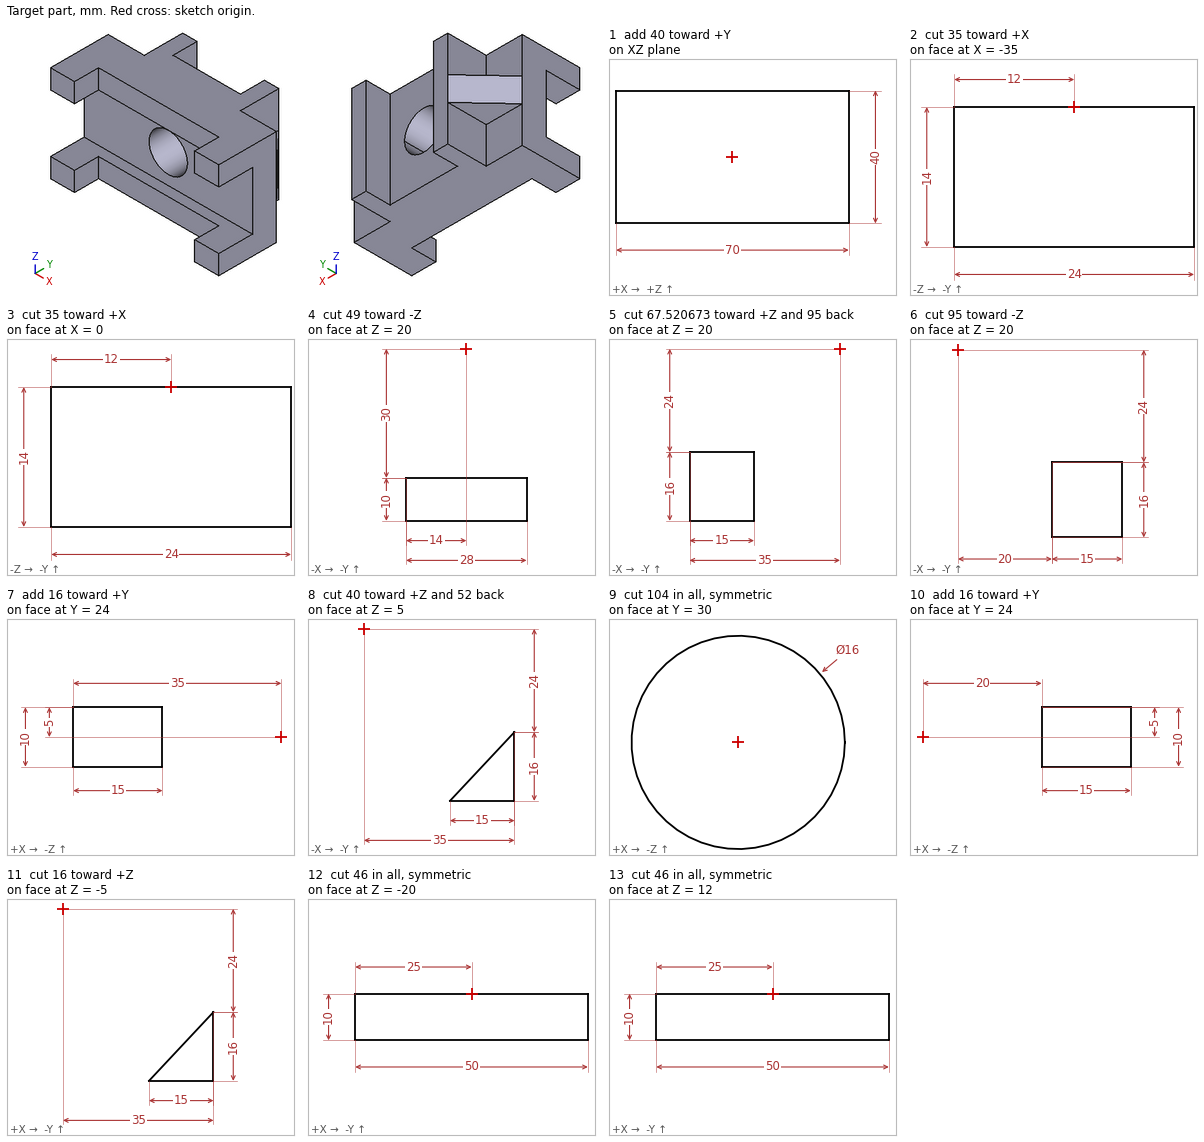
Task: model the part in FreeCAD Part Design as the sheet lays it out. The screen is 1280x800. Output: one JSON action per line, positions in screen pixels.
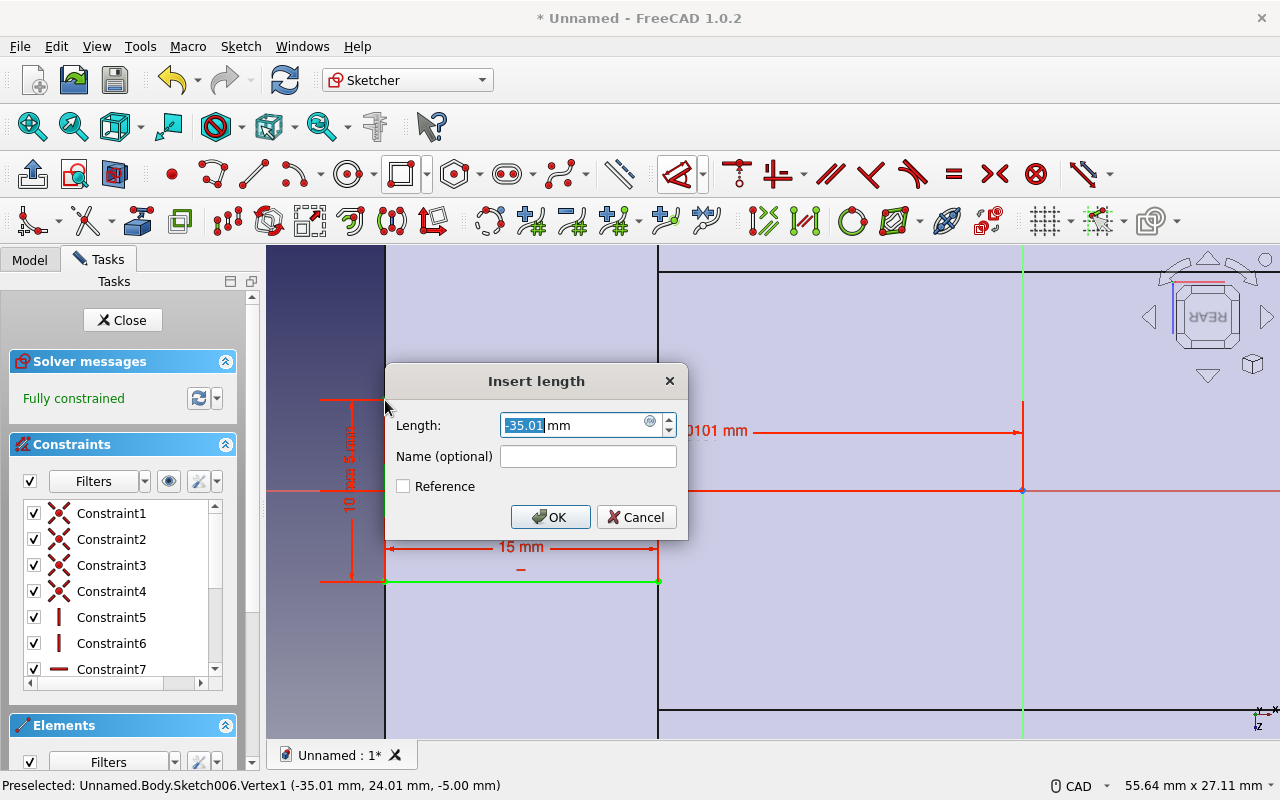
{"action": "type", "text": "-35"}
{"action": "key", "text": "Return"}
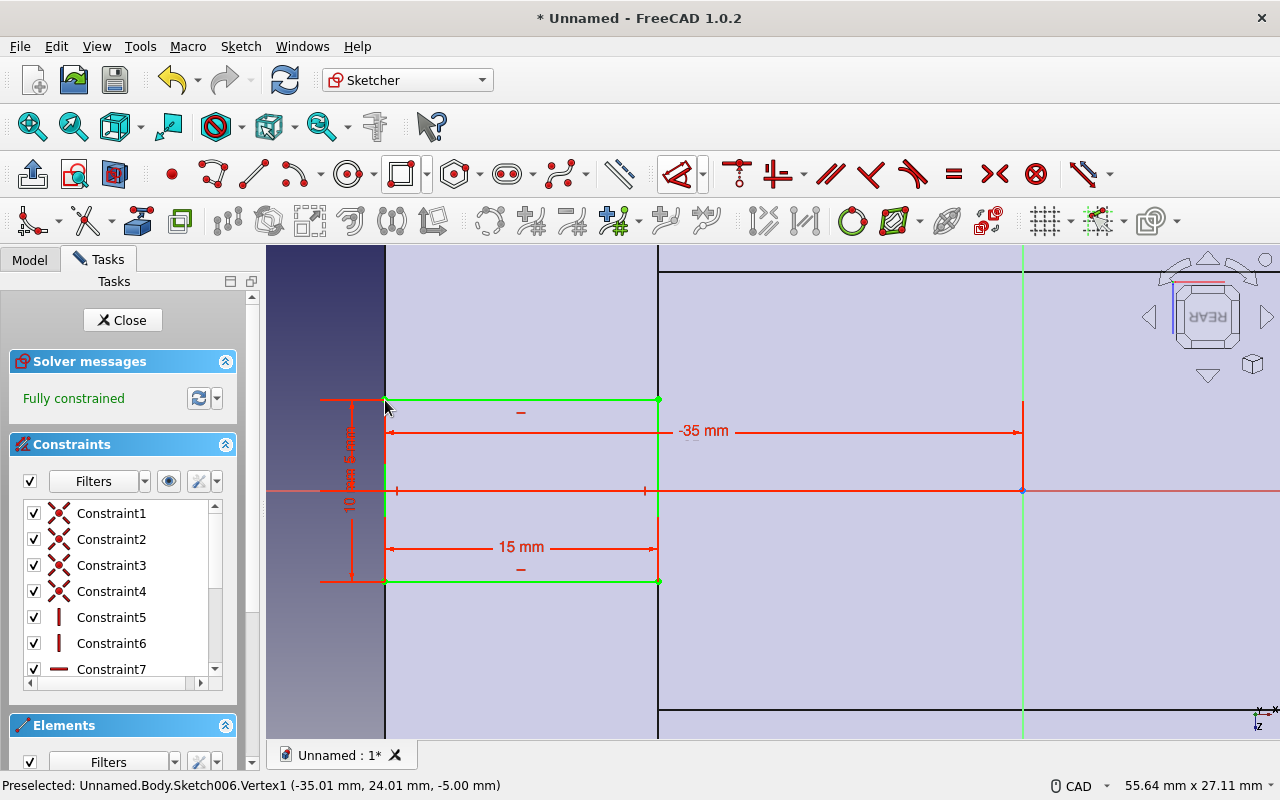
{"action": "left_click", "coordinate": [123, 320]}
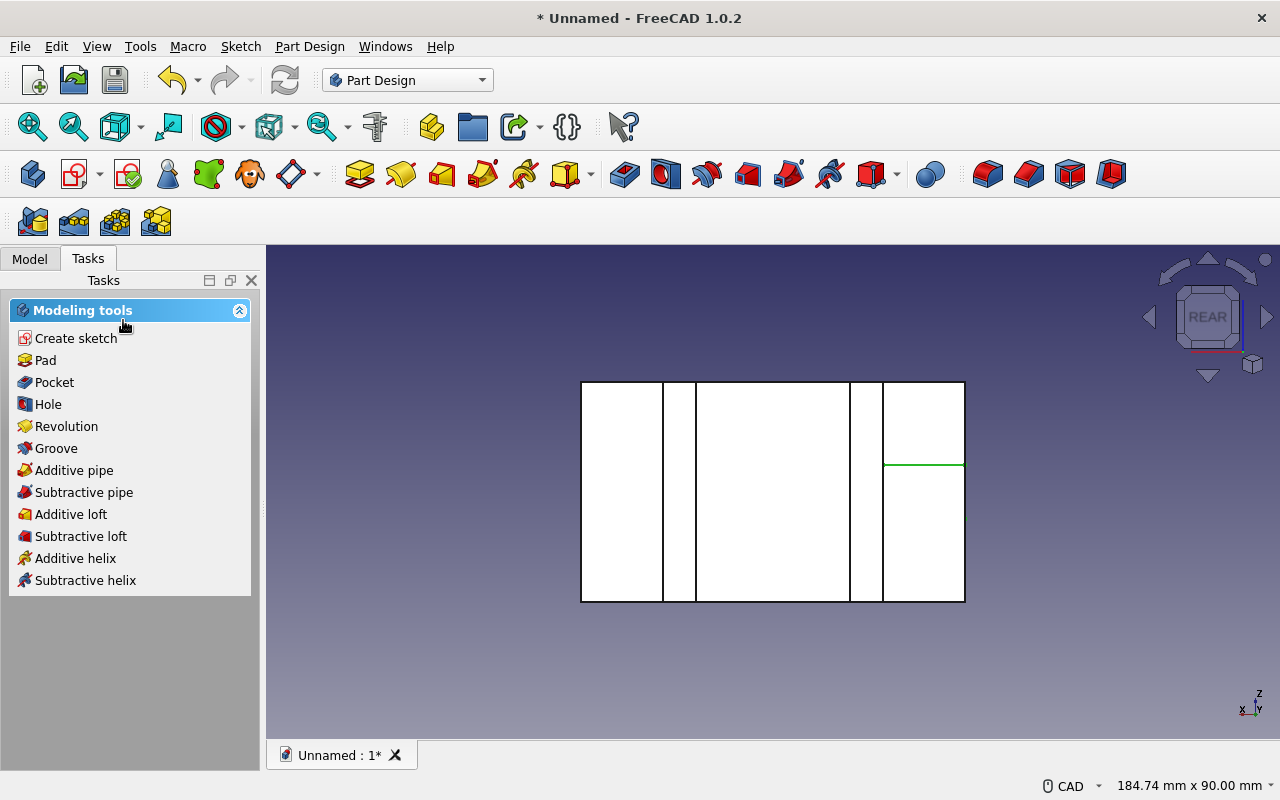
{"action": "left_click", "coordinate": [360, 174]}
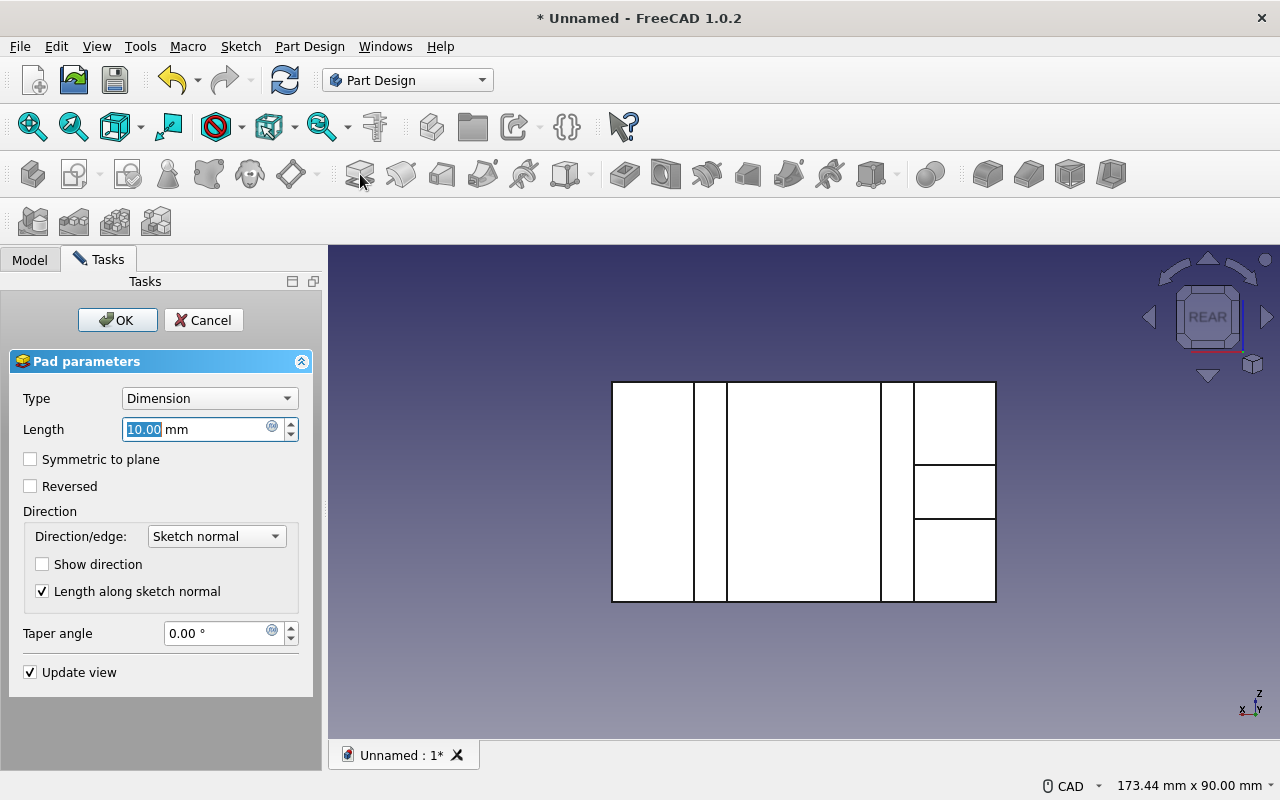
{"action": "type", "text": "16"}
{"action": "key", "text": "Tab"}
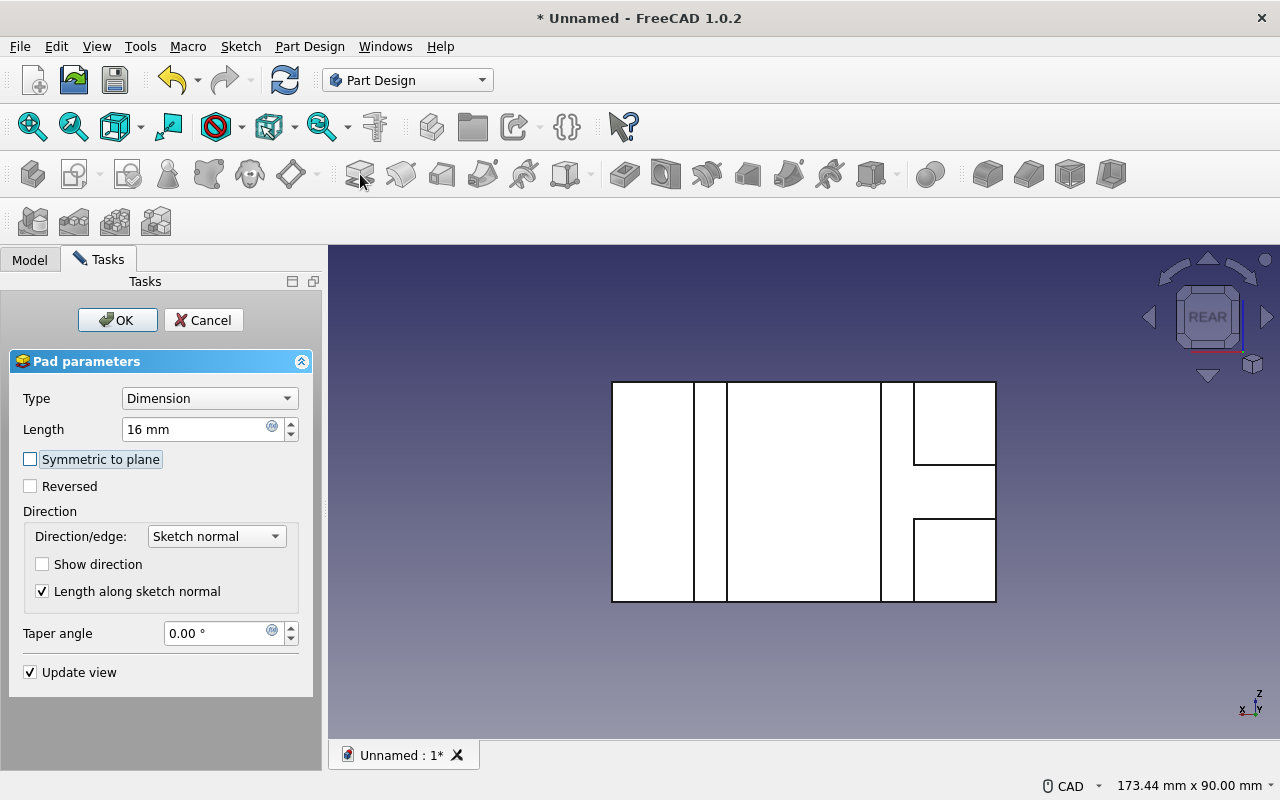
{"action": "left_click", "coordinate": [118, 320]}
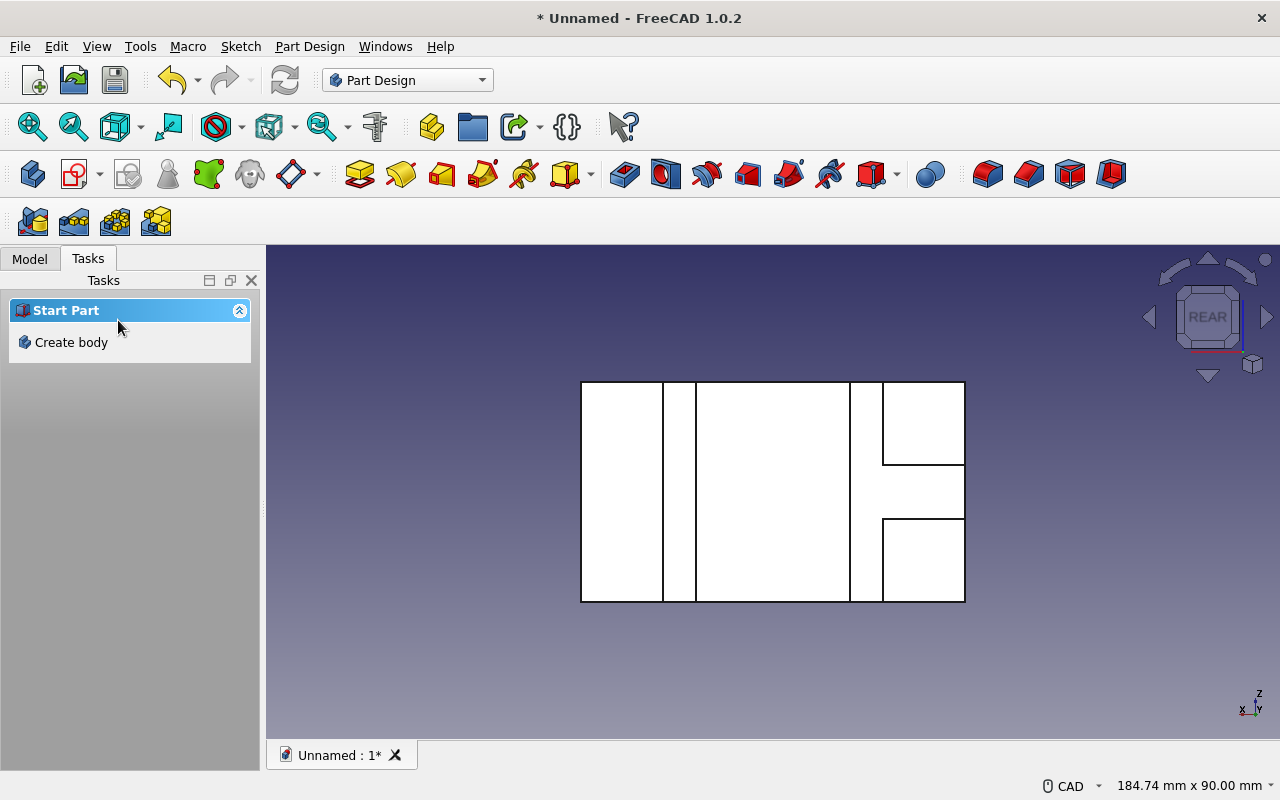
{"action": "key", "text": "v f"}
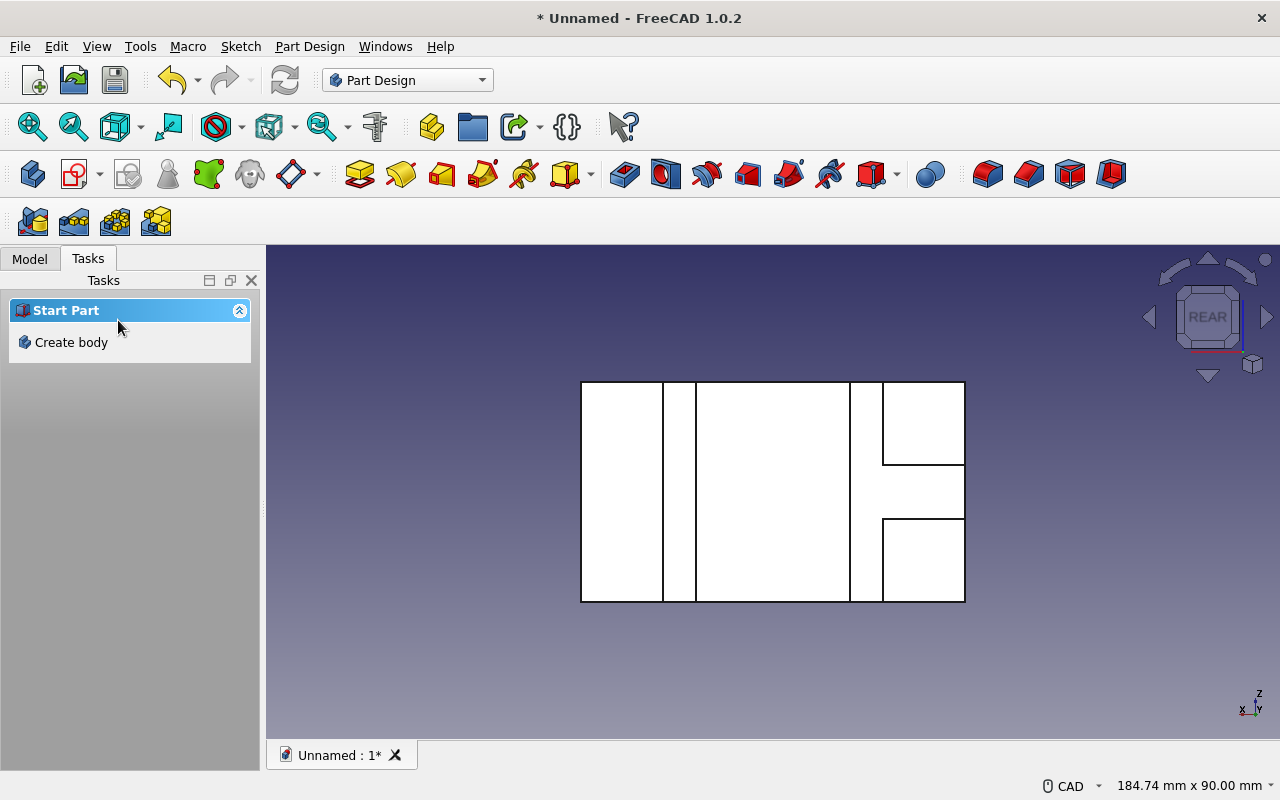
{"action": "key", "text": "0"}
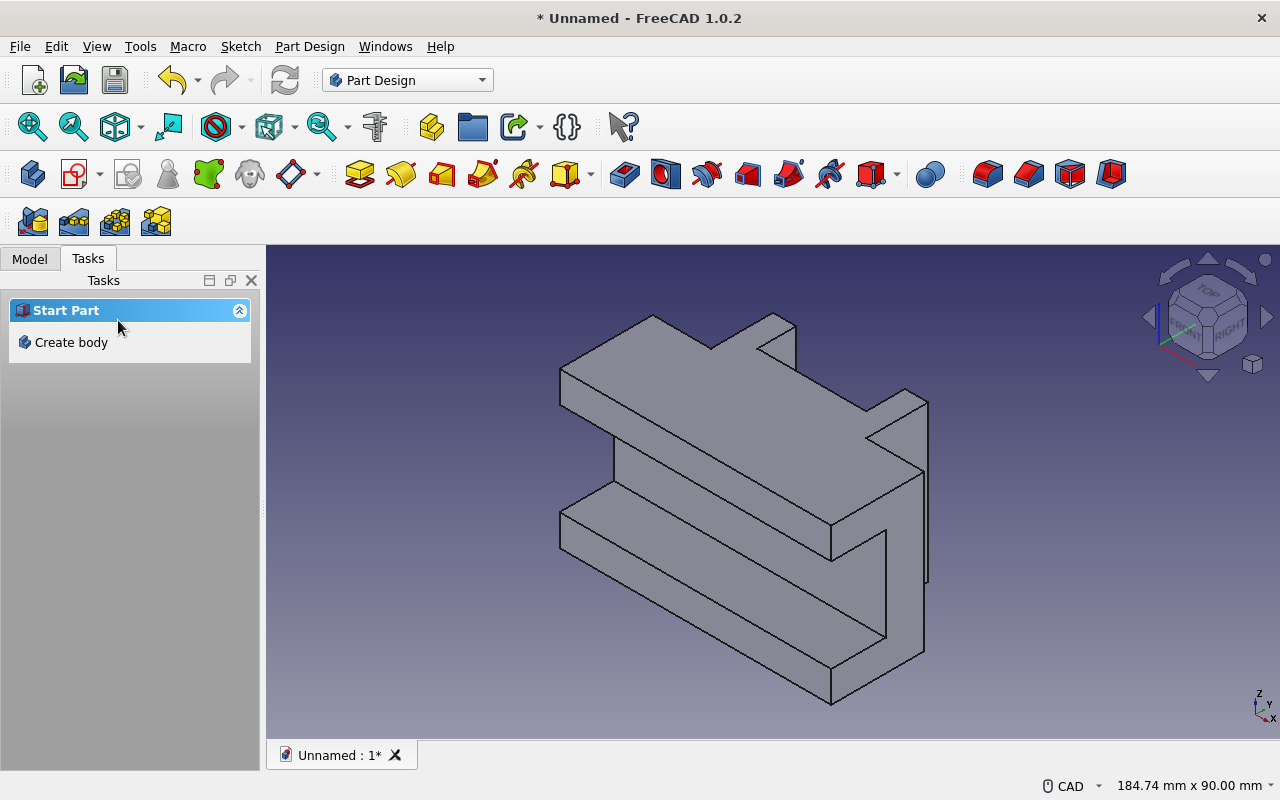
{"action": "key", "text": "2"}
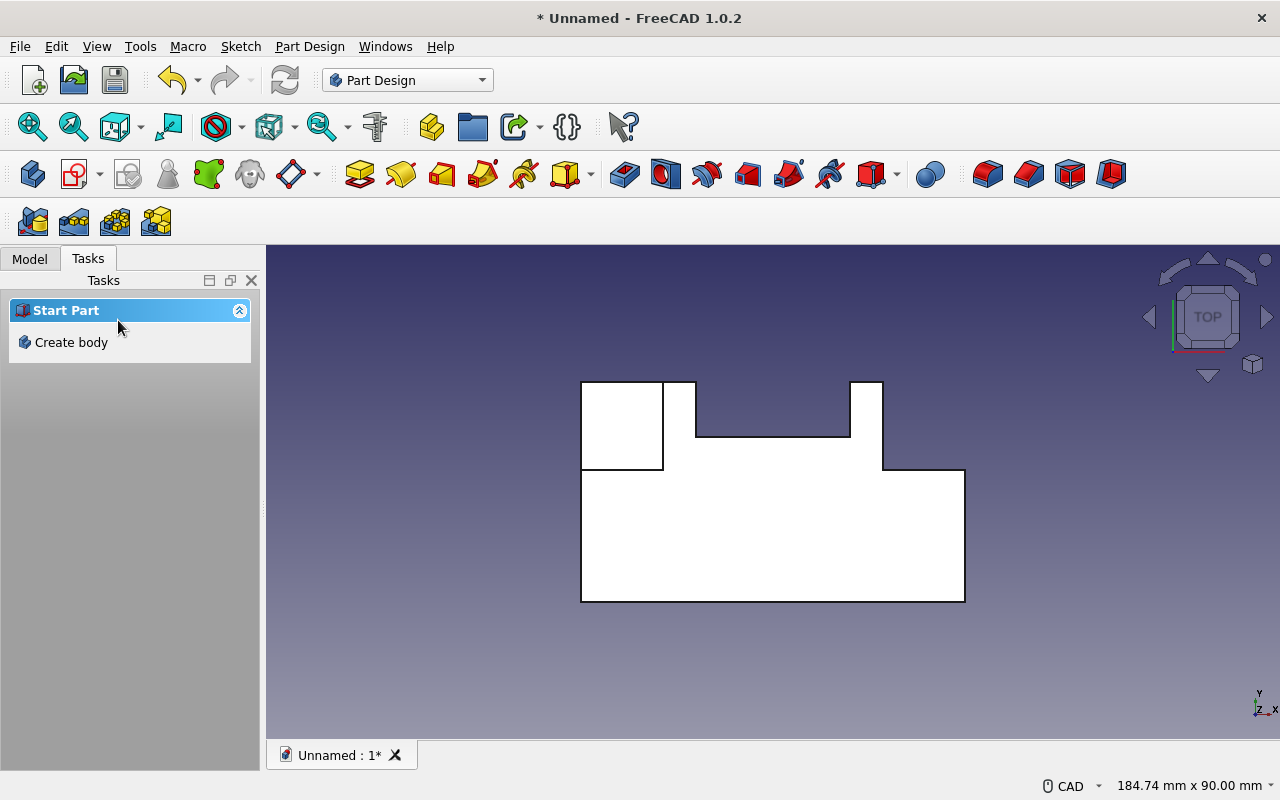
{"action": "left_click", "coordinate": [33, 128]}